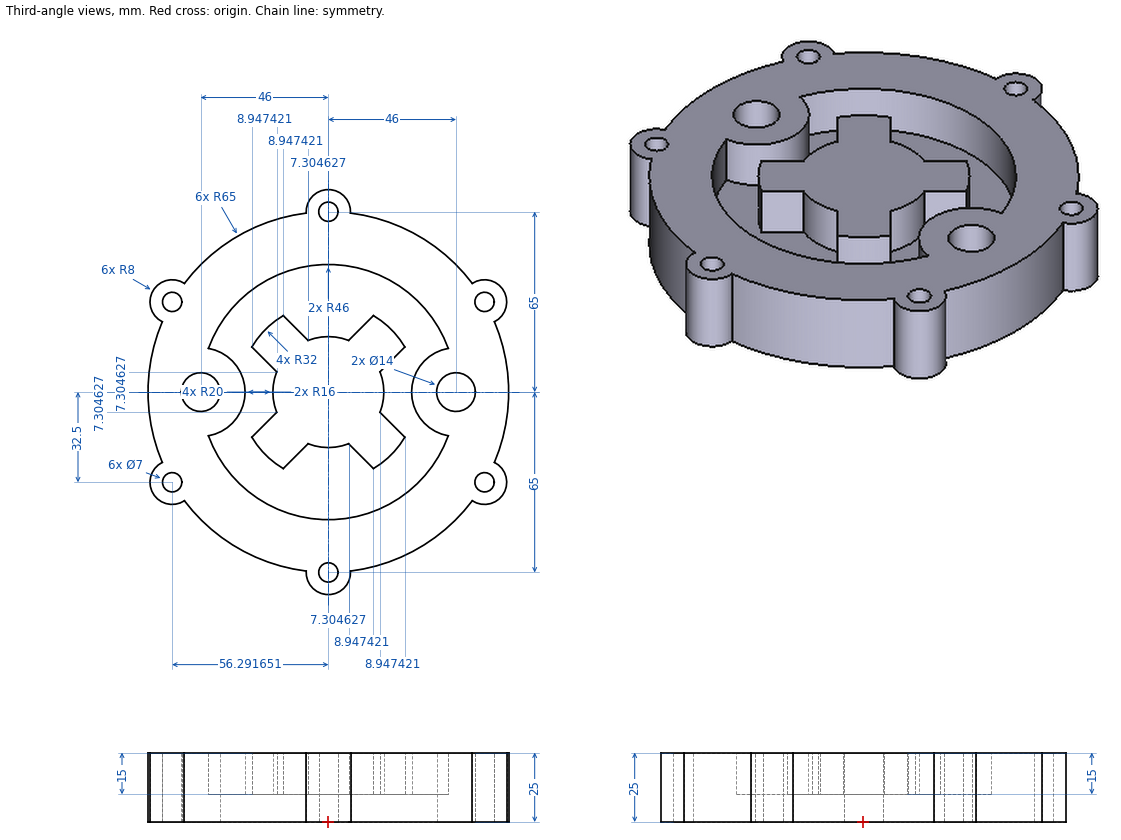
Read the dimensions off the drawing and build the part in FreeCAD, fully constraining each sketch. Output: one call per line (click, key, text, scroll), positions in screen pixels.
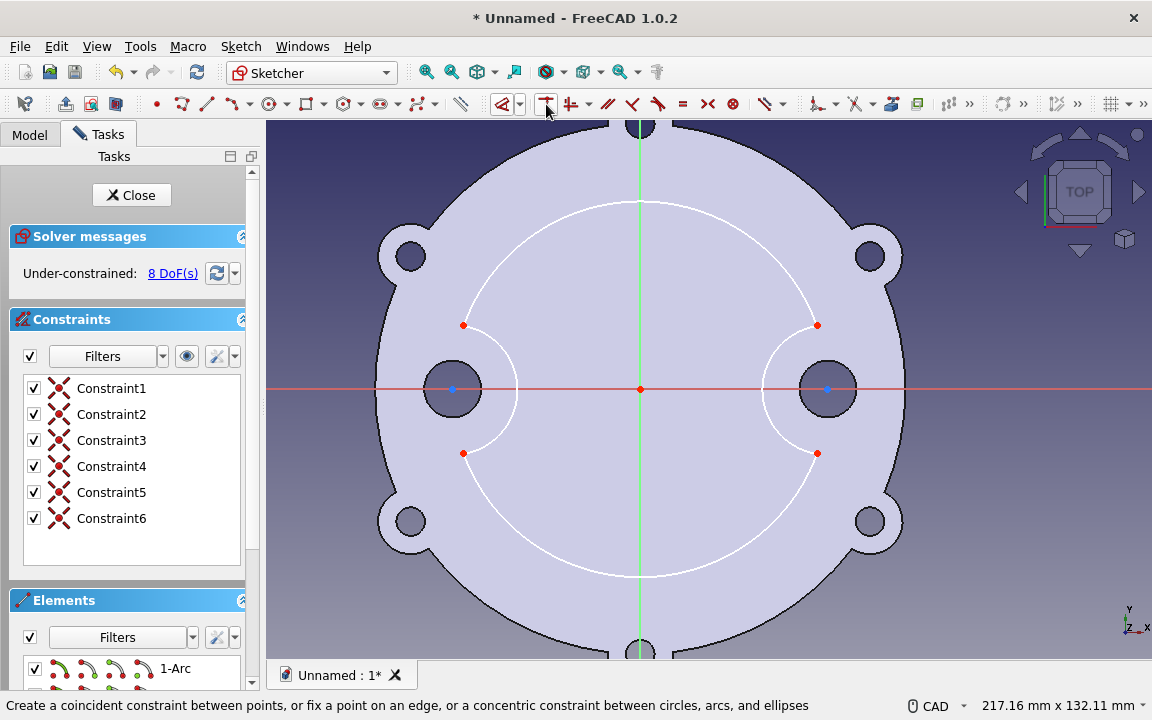
click(729, 224)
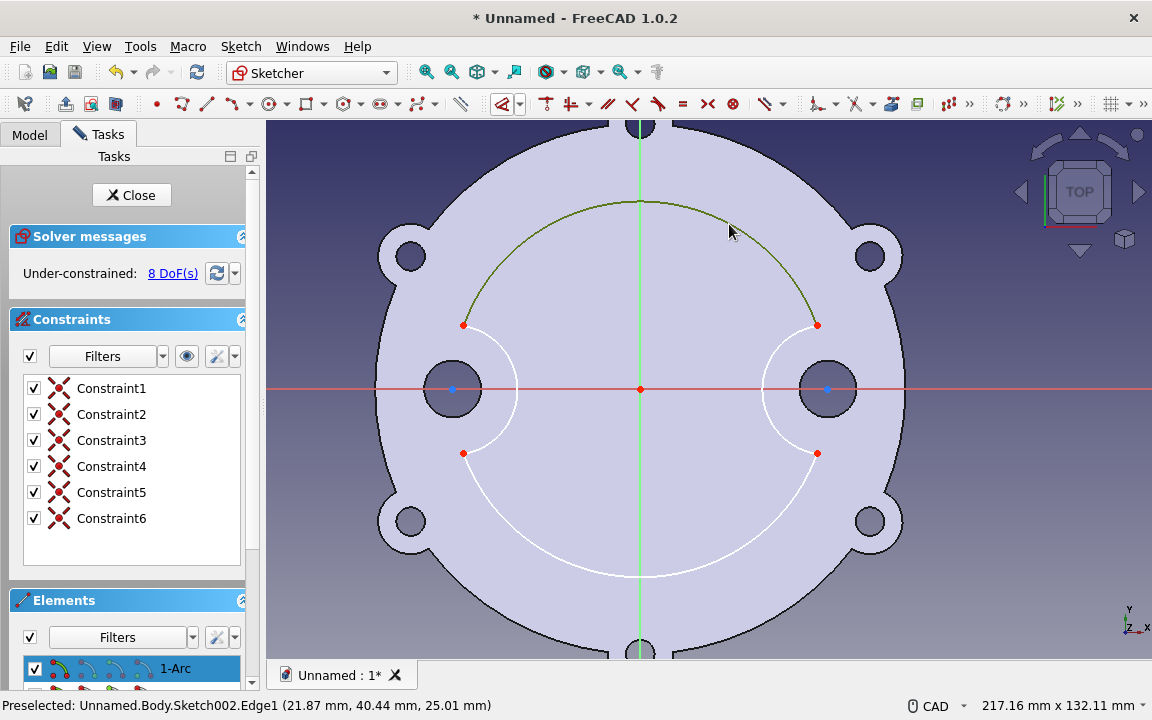
click(552, 555)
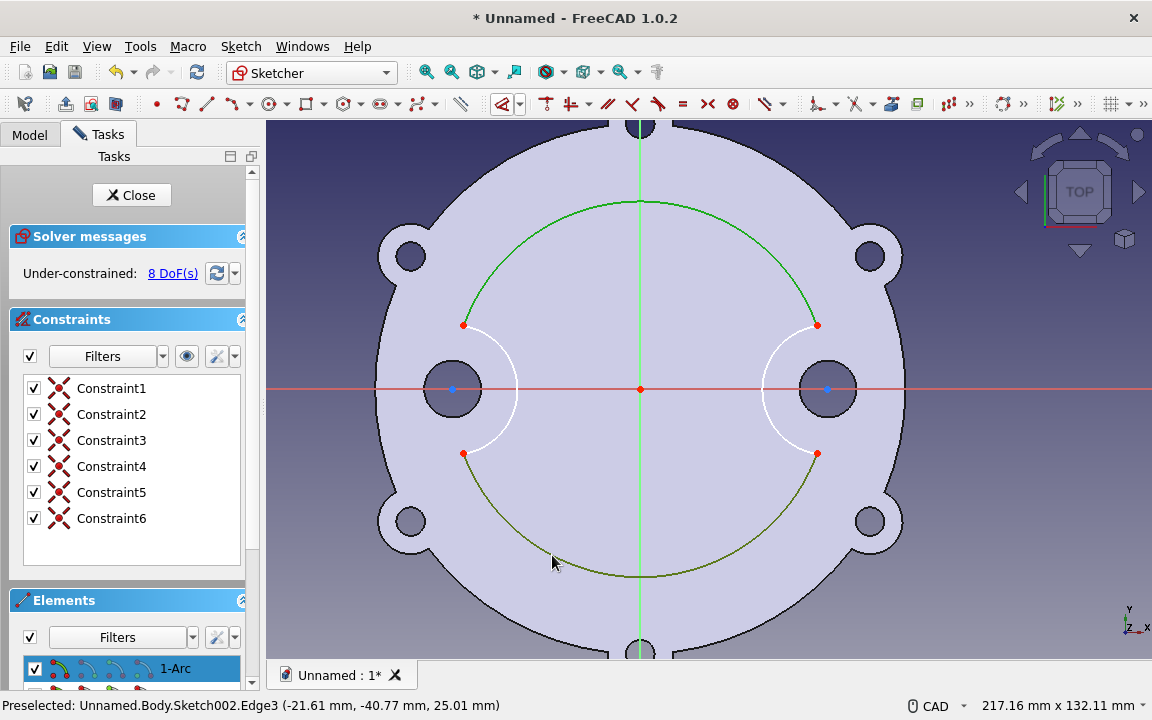
click(683, 104)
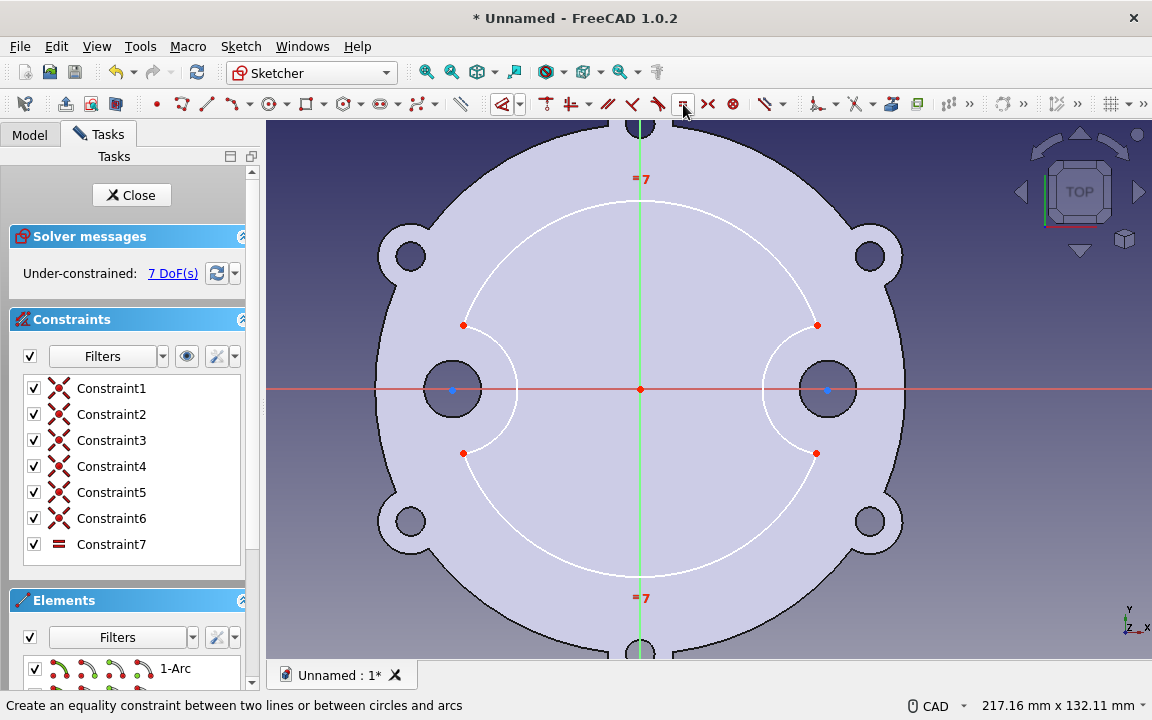
click(508, 424)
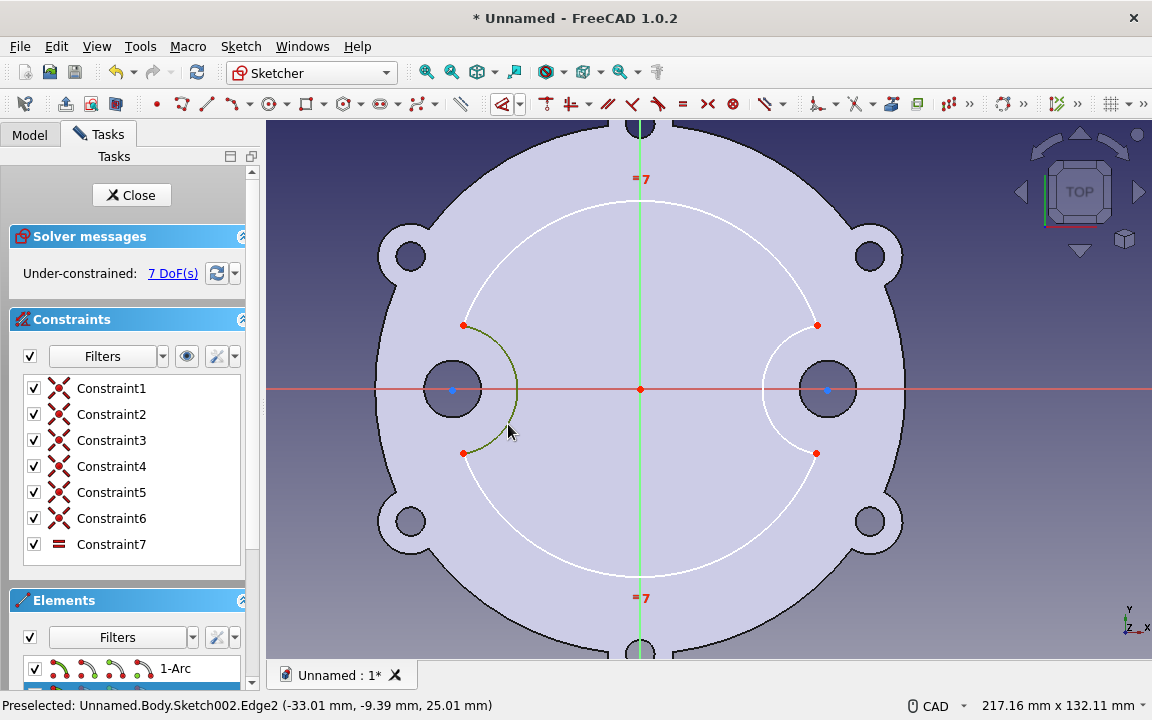
click(773, 355)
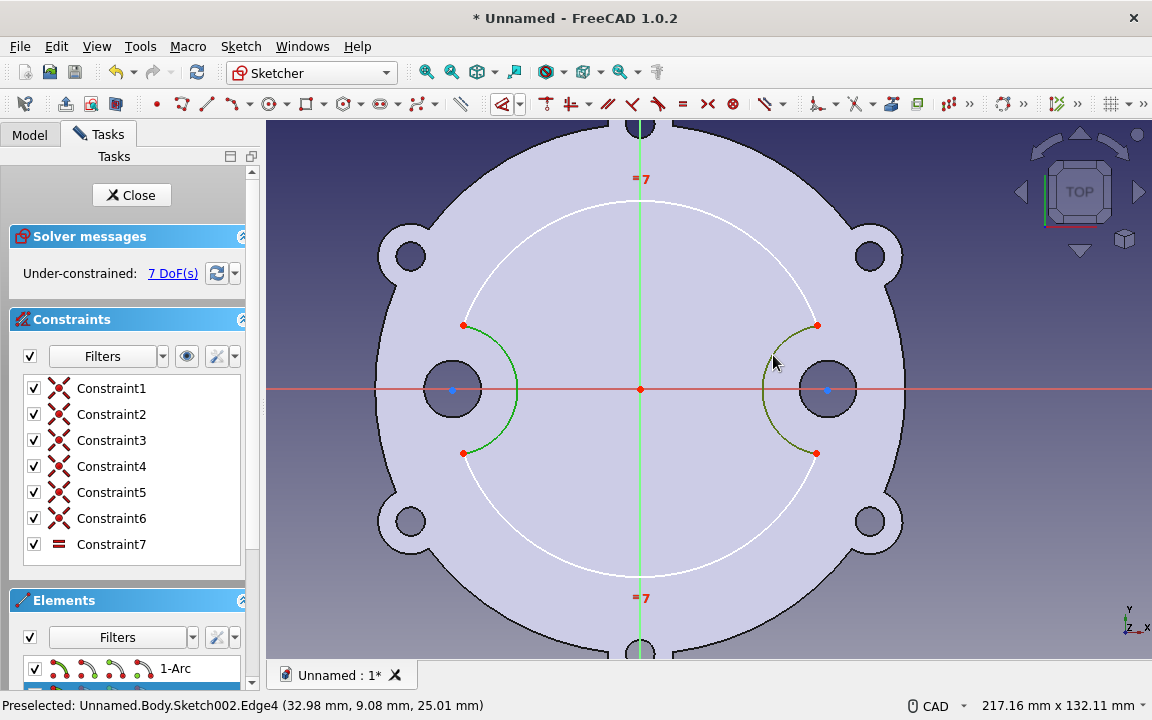
click(683, 104)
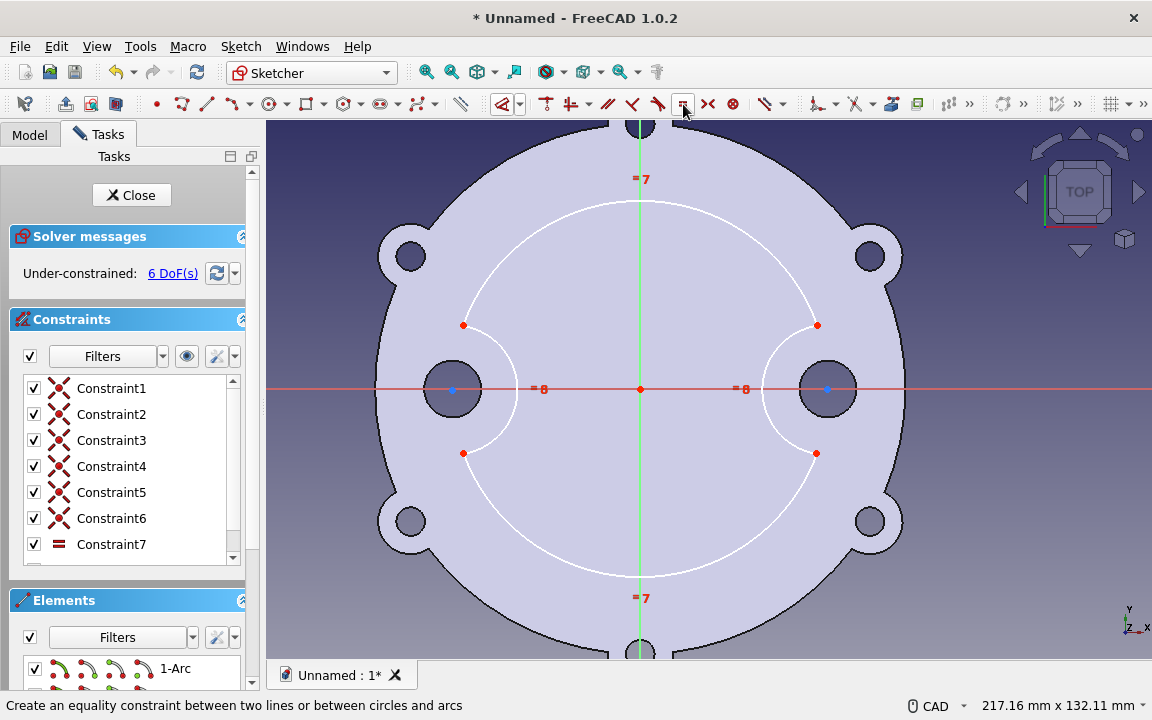
click(453, 390)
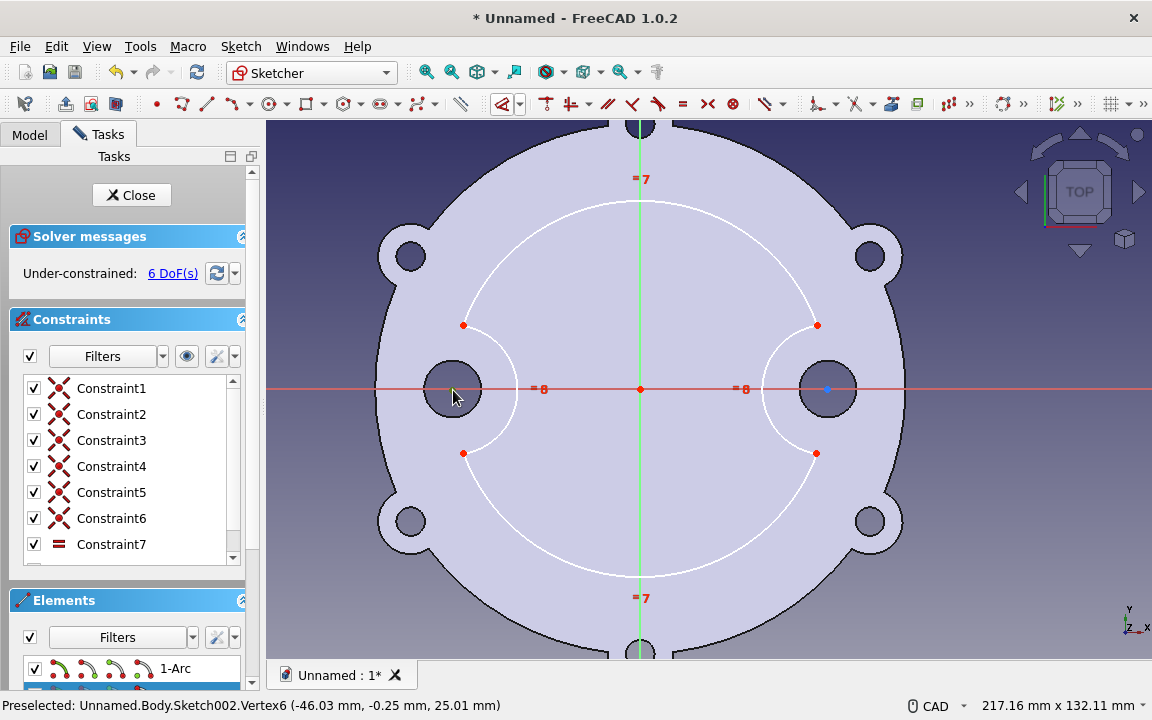
click(344, 389)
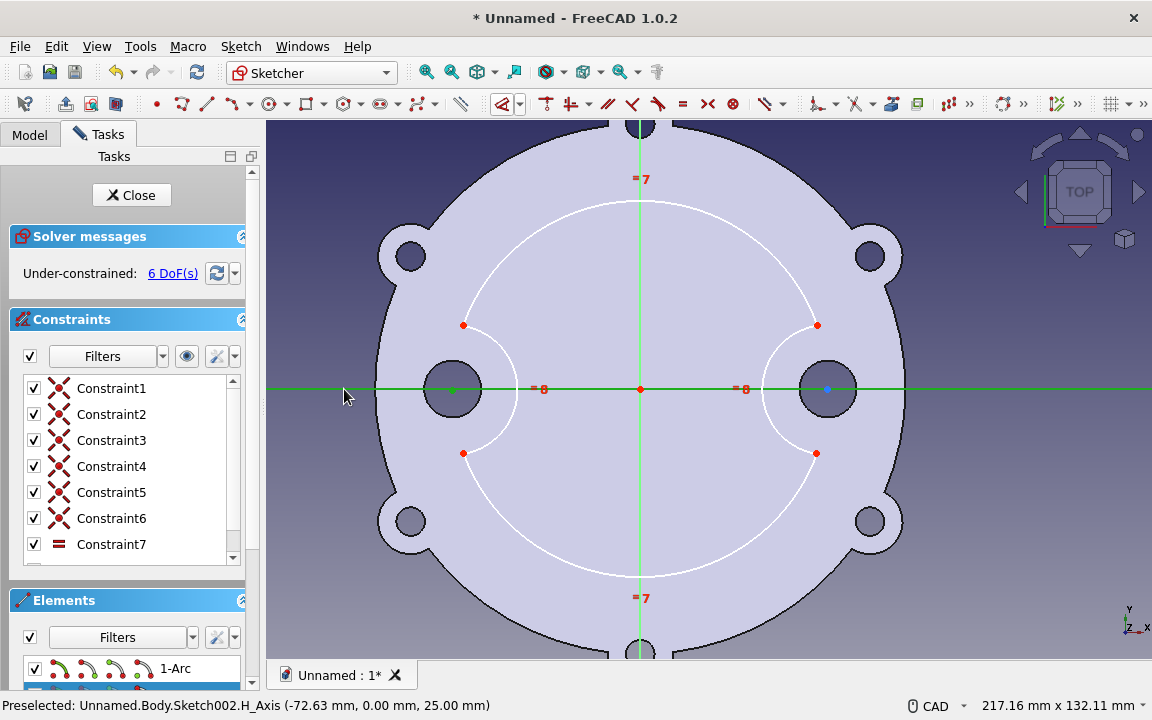
click(546, 104)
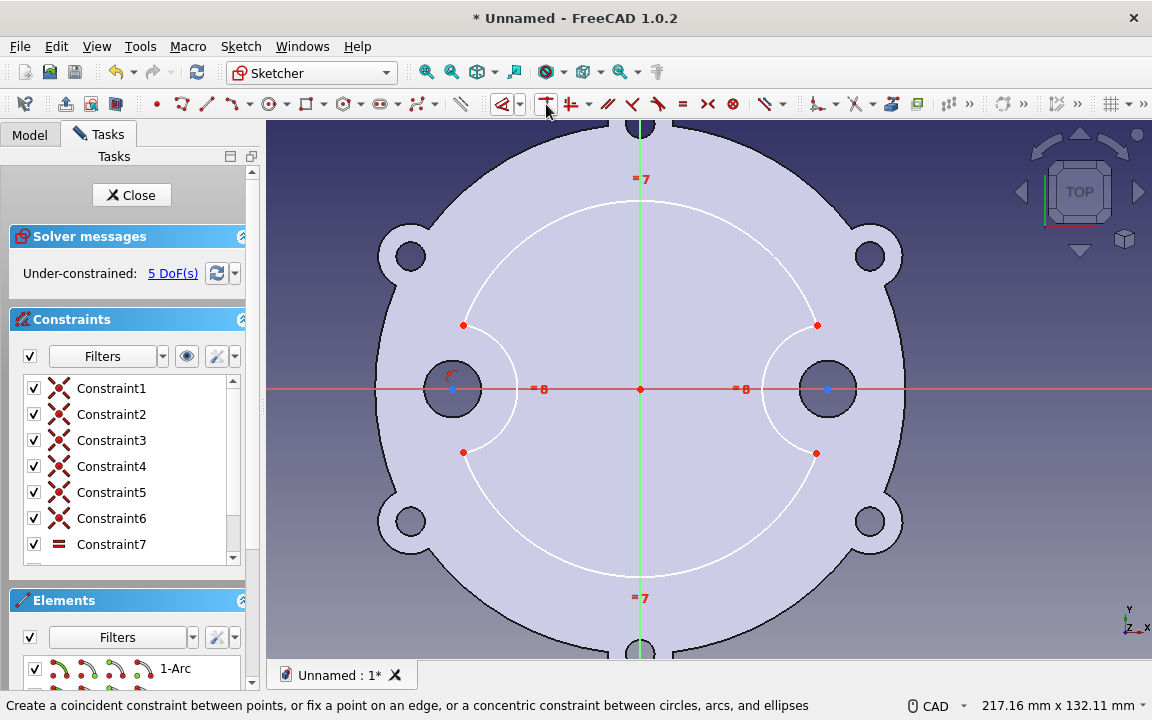
click(827, 390)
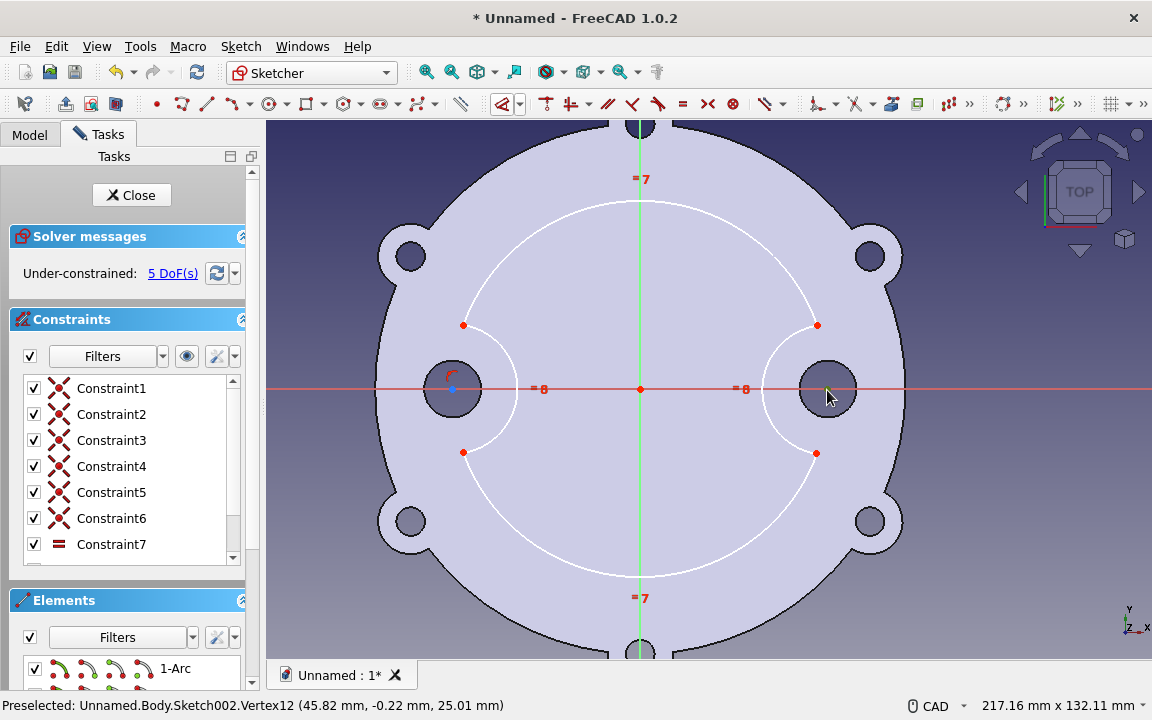
click(344, 389)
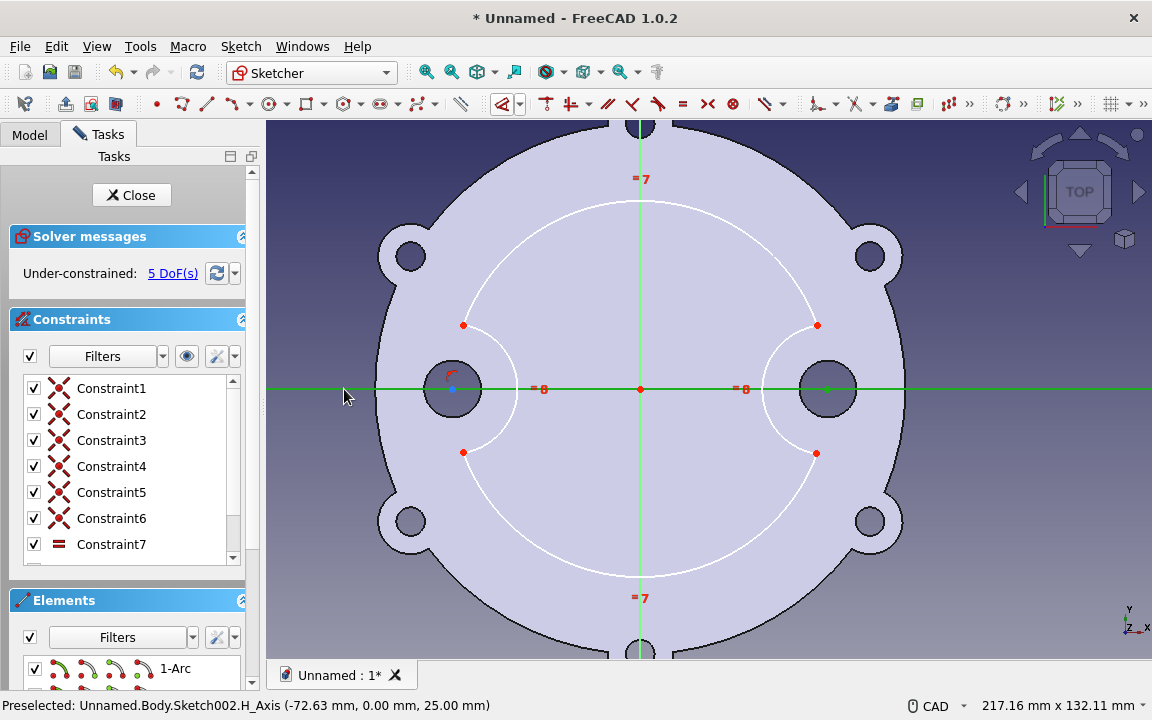
click(546, 104)